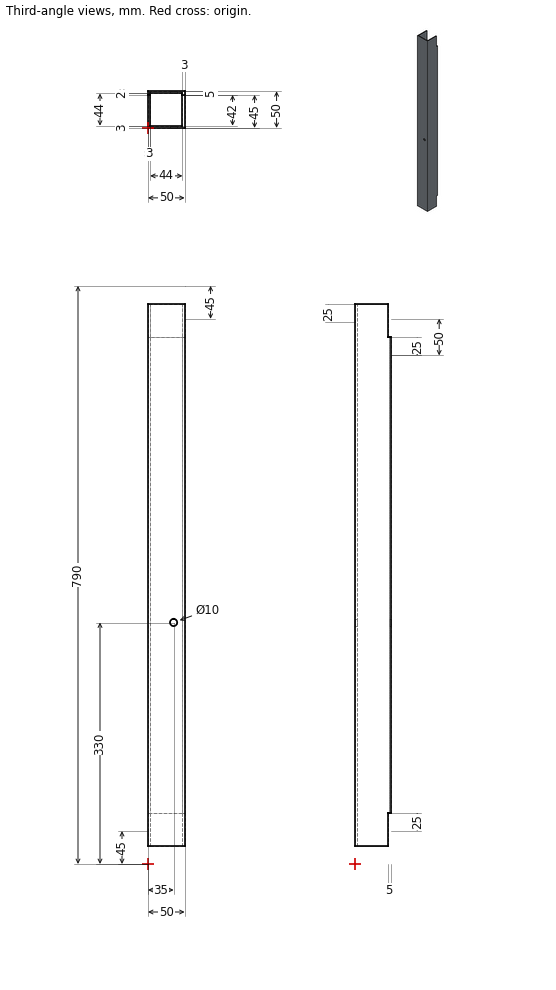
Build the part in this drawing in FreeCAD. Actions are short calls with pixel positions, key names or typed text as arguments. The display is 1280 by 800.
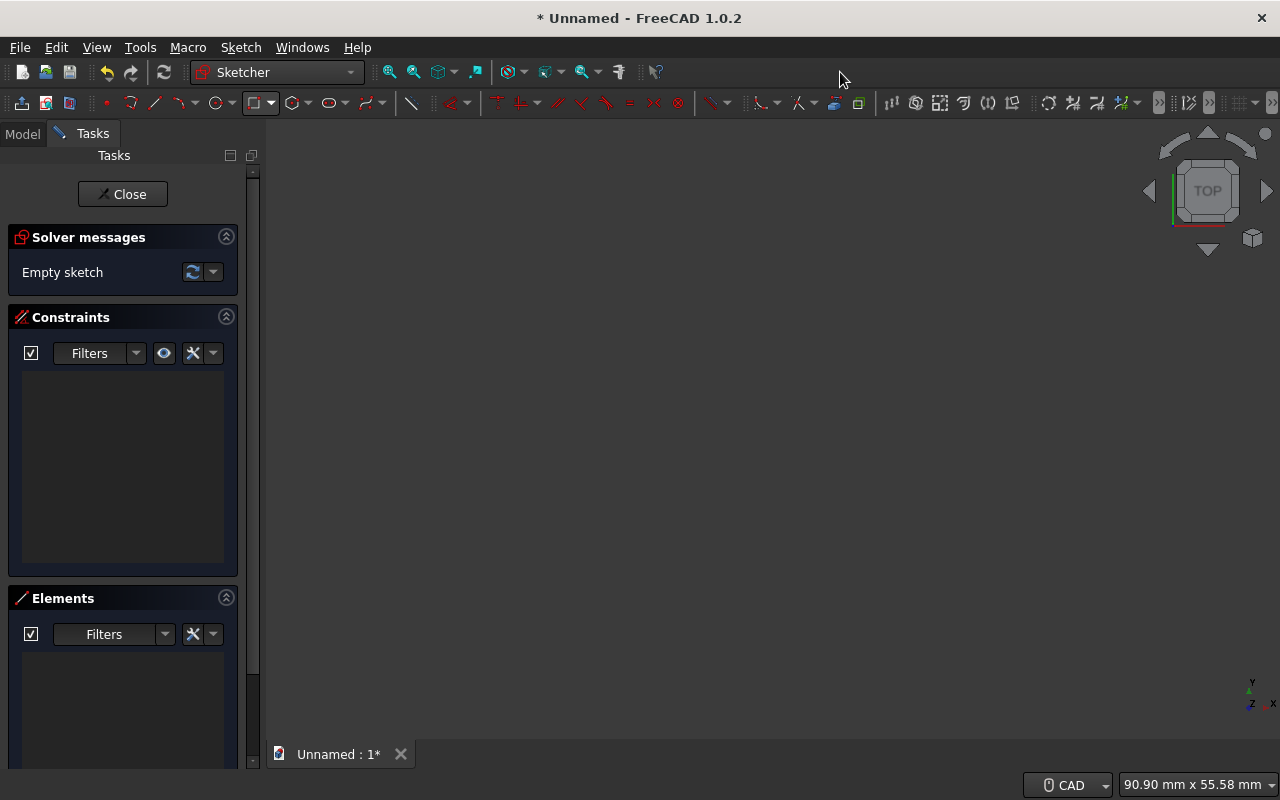
scroll(704, 429, down, 5)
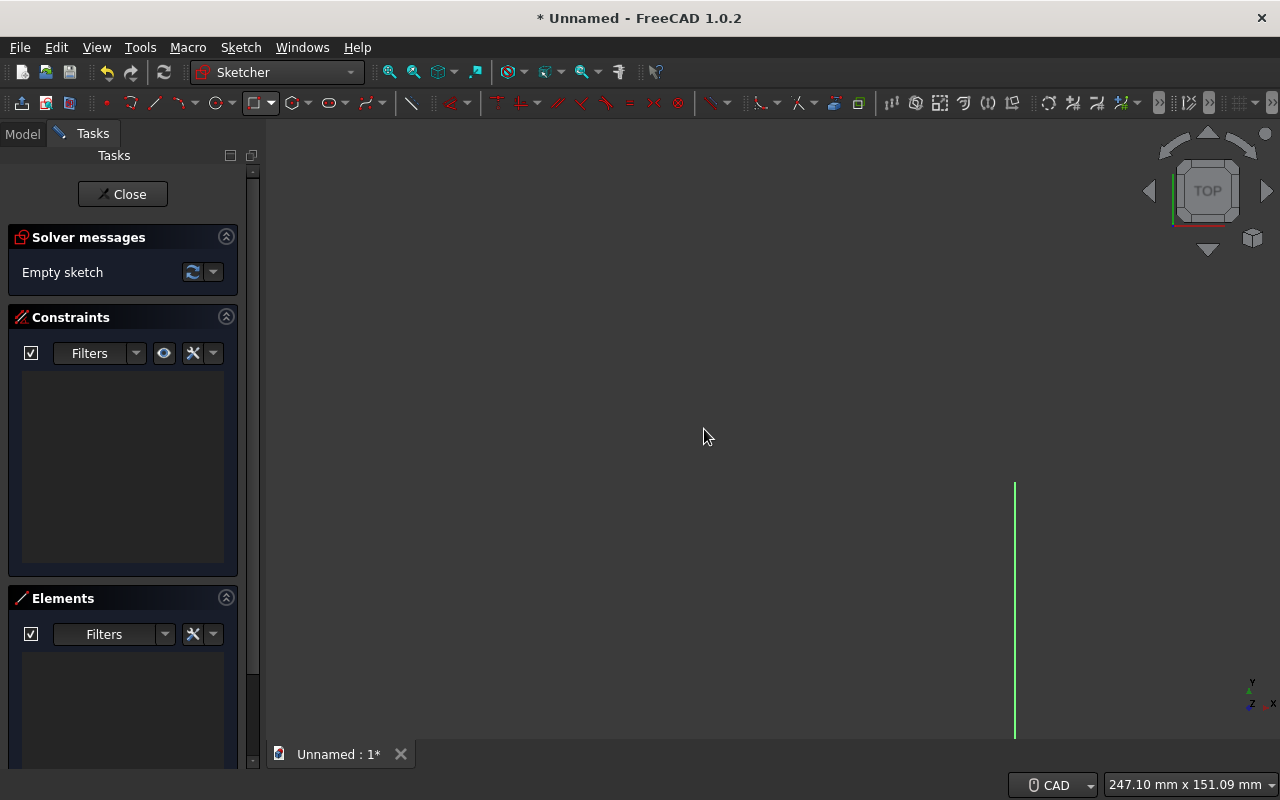
scroll(704, 429, down, 5)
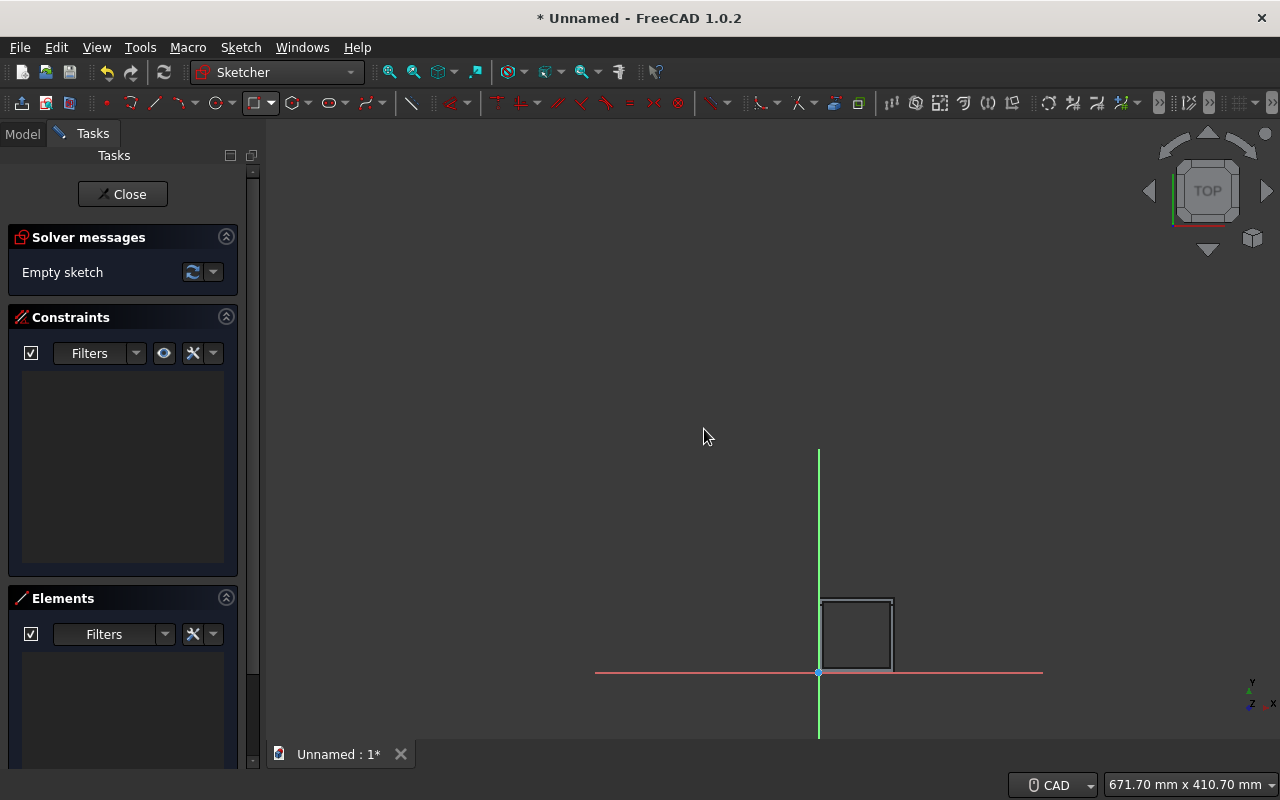
scroll(895, 687, up, 8)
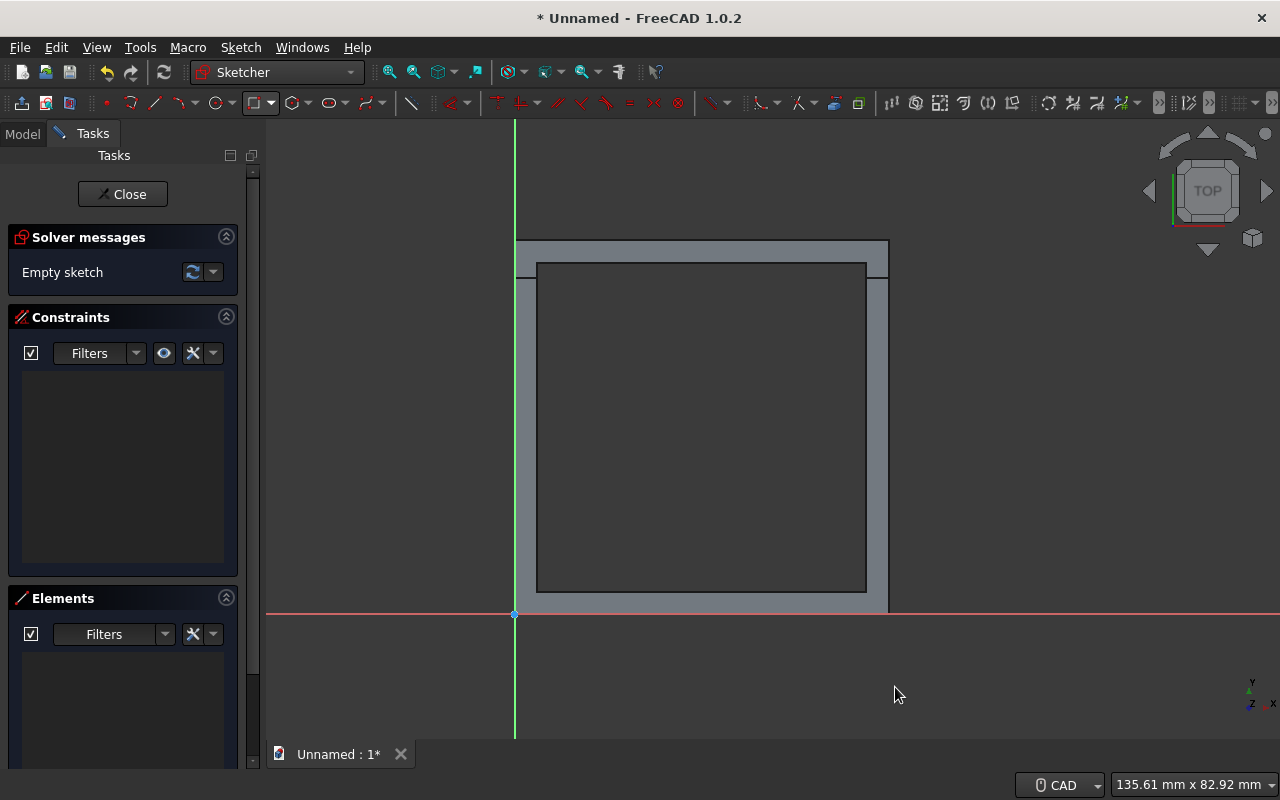
click(132, 104)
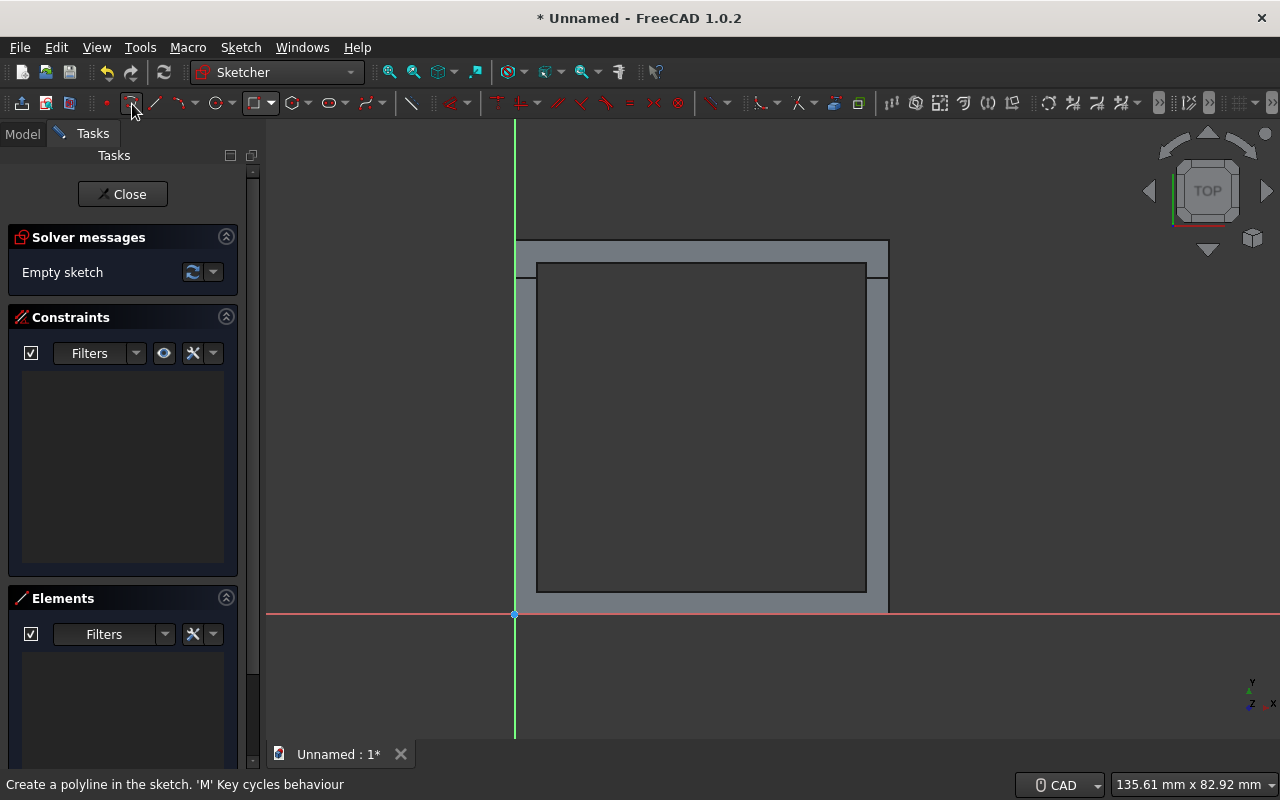
click(515, 278)
click(537, 278)
click(537, 263)
click(866, 263)
click(866, 278)
click(889, 278)
click(889, 240)
click(524, 240)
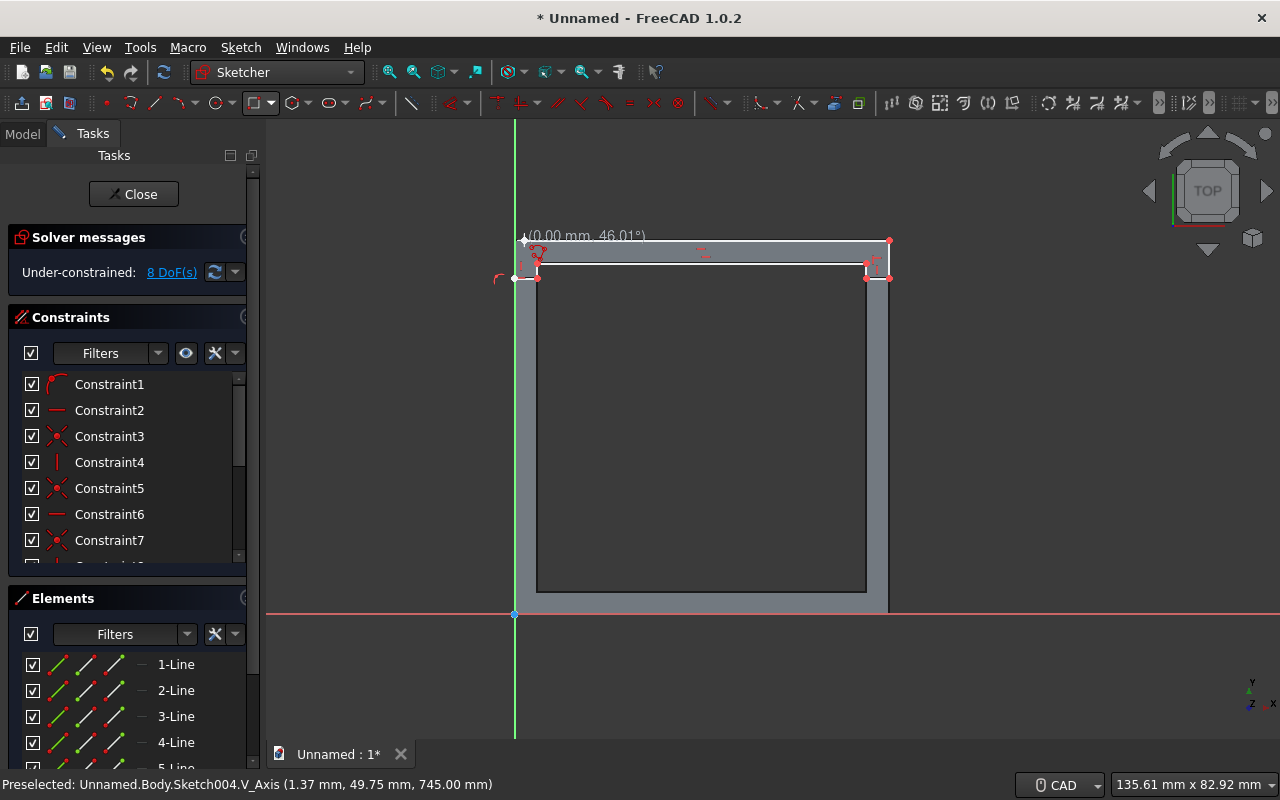
scroll(515, 278, up, 2)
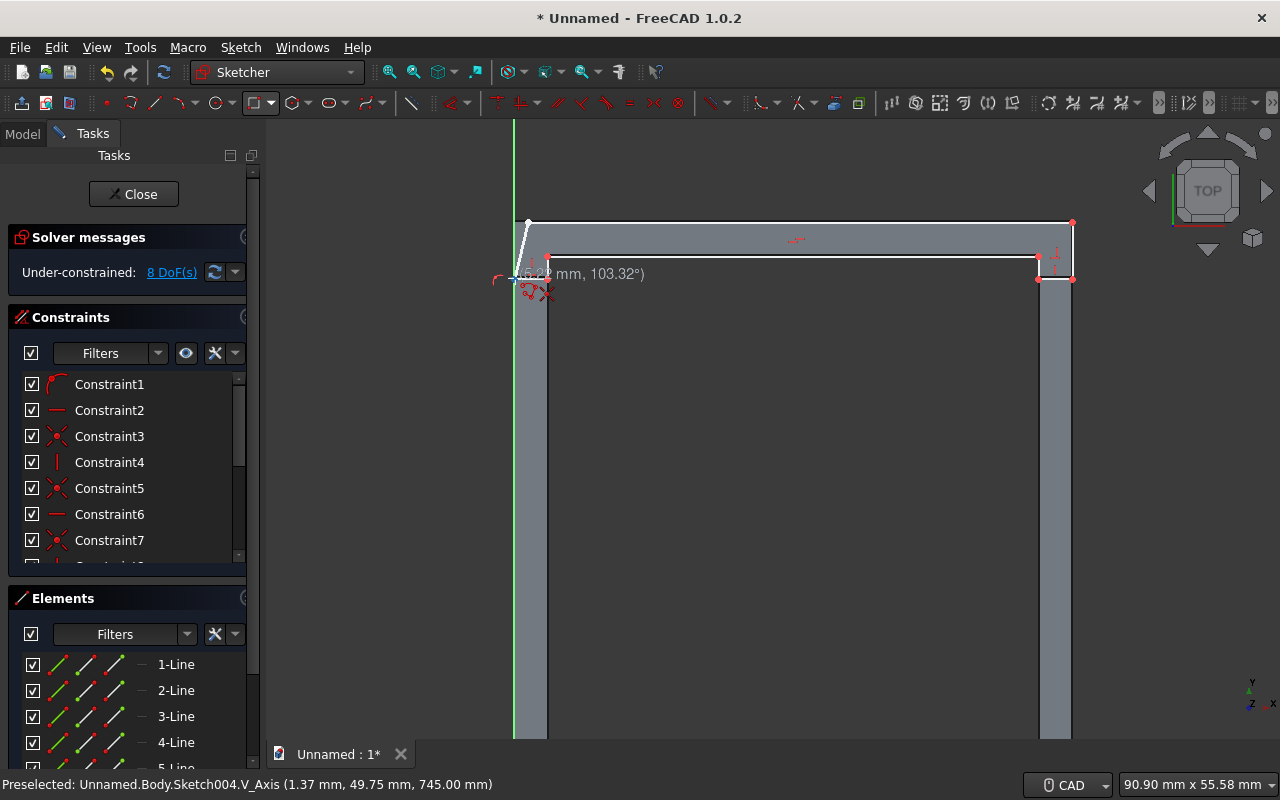
click(514, 279)
key(Escape)
key(Escape)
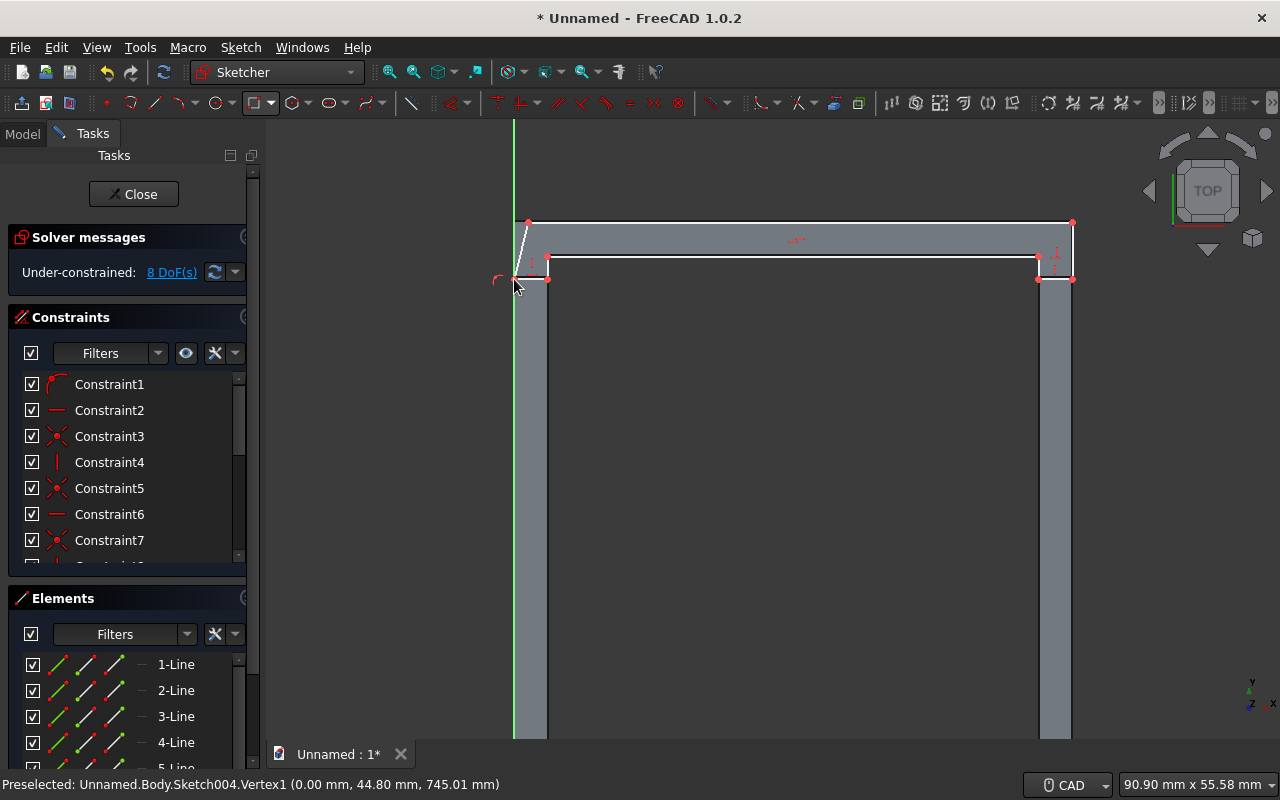
scroll(524, 240, up, 2)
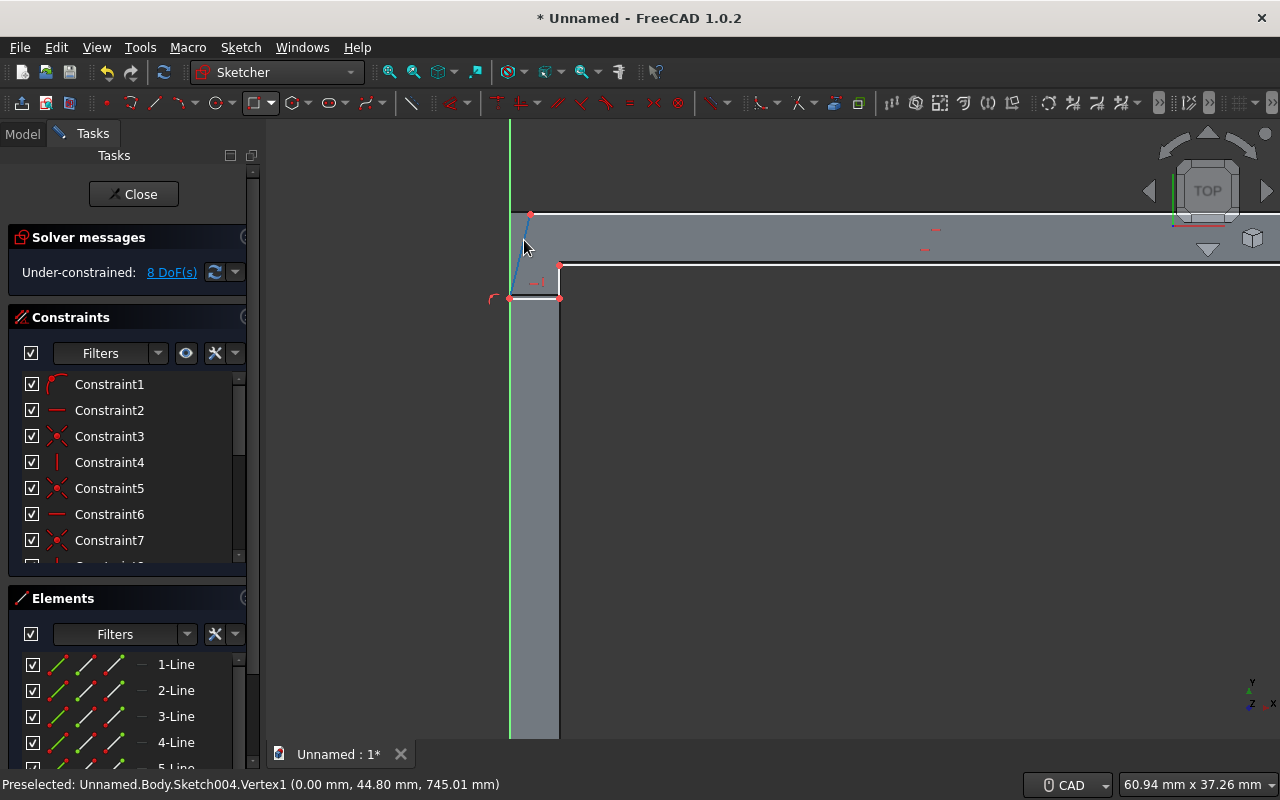
click(524, 239)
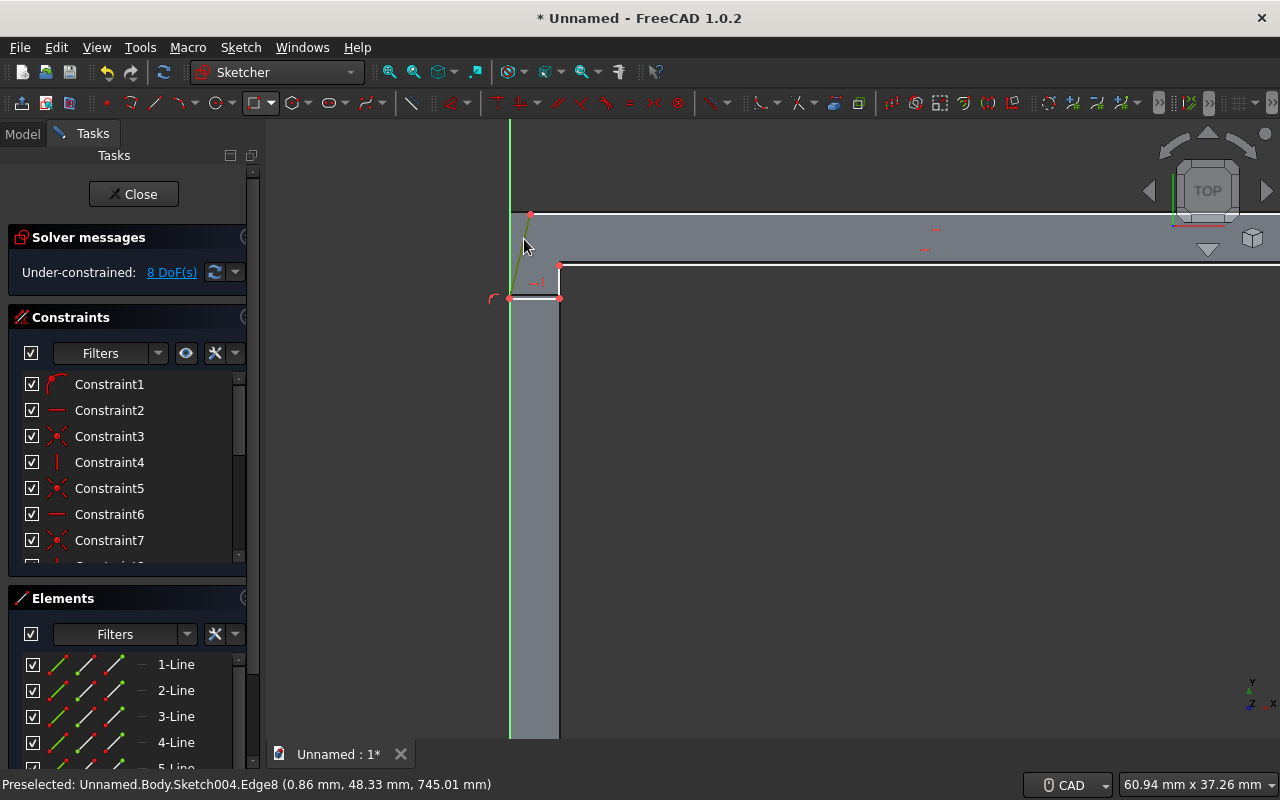
click(540, 104)